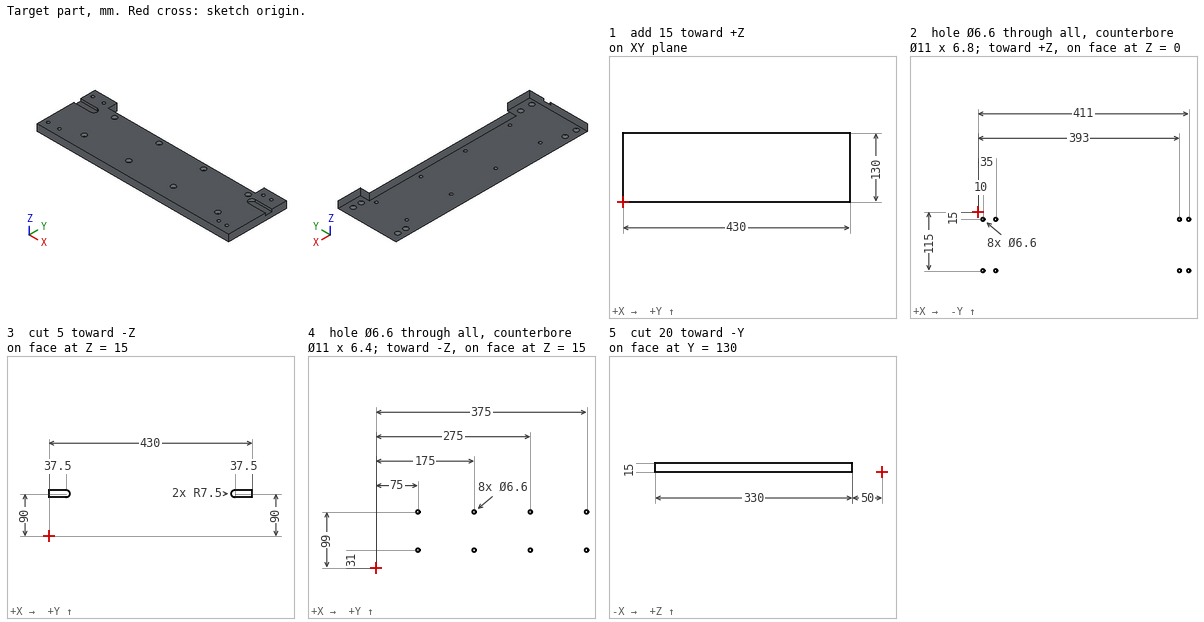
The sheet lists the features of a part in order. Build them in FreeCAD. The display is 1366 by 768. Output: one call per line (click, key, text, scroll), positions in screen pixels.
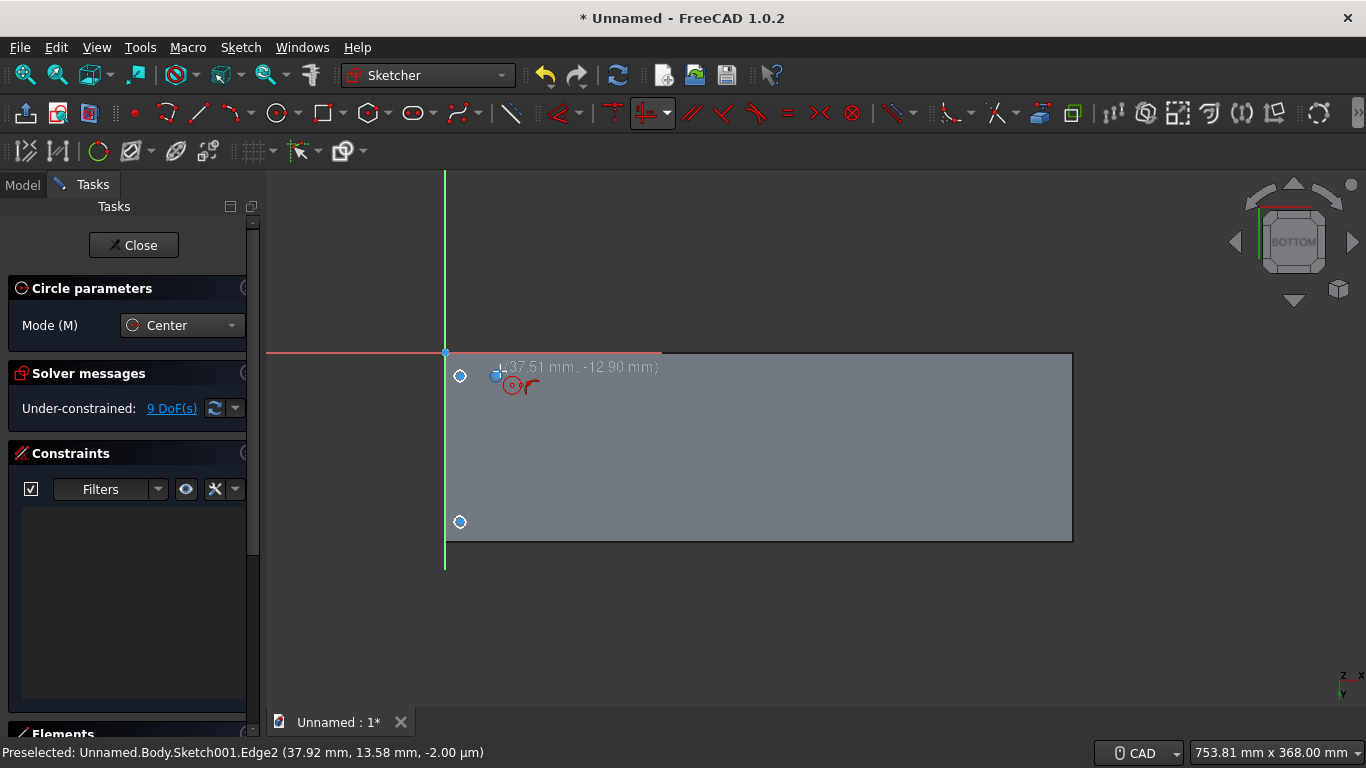
scroll(496, 521, up, 8)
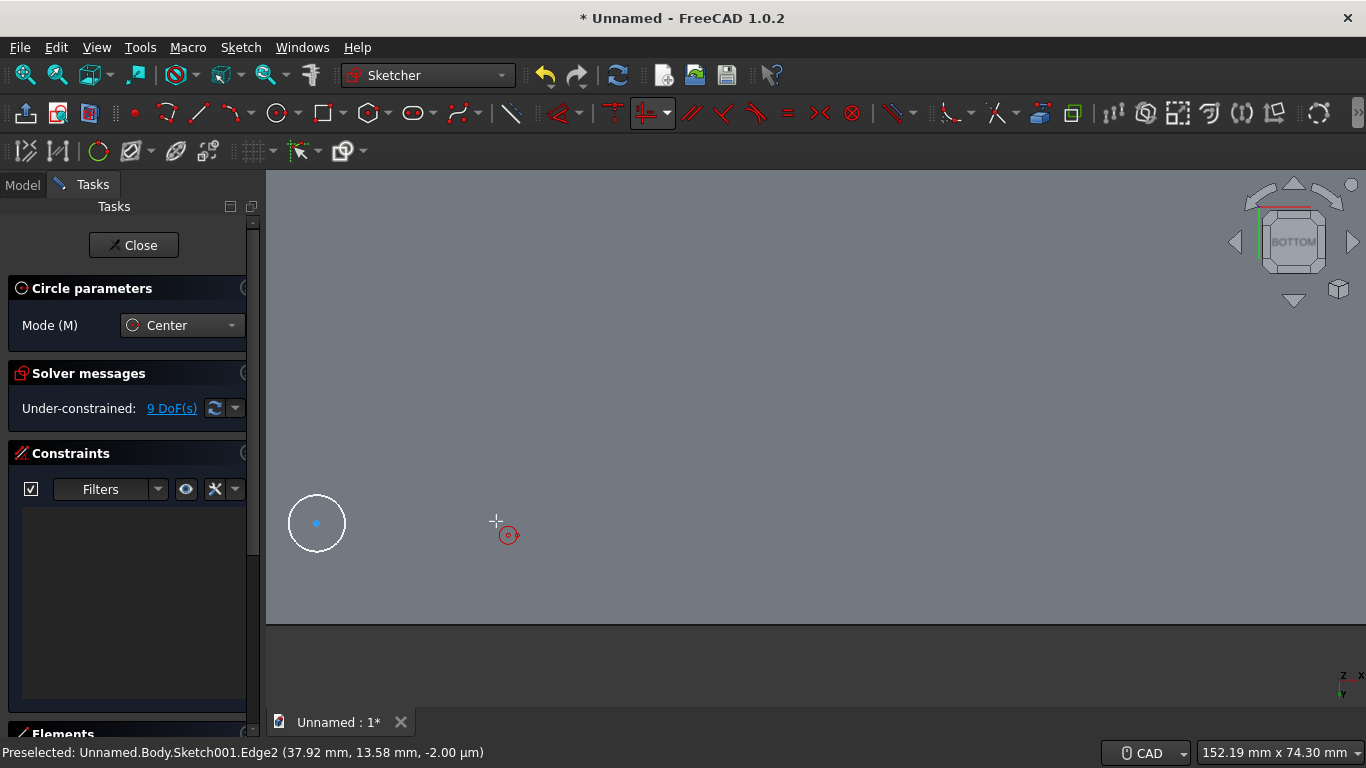
scroll(496, 521, down, 8)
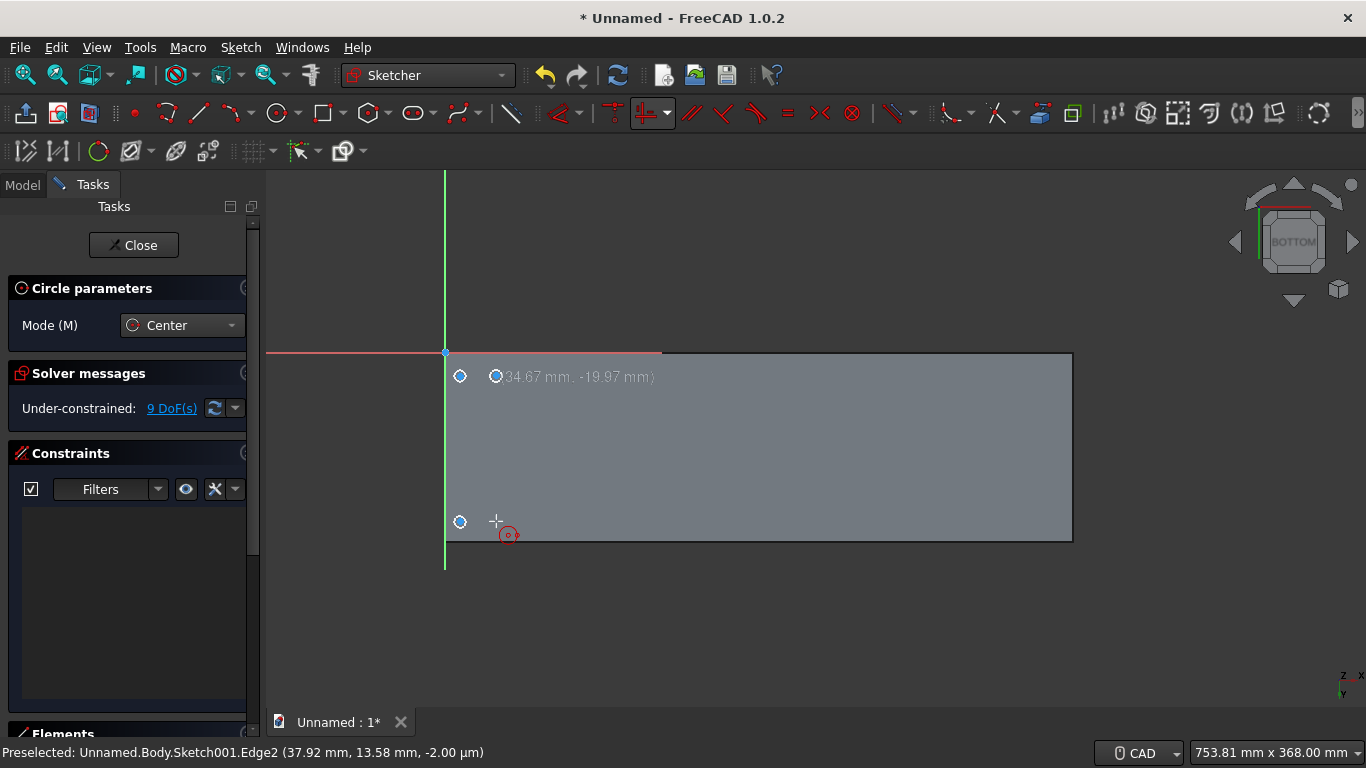
click(496, 521)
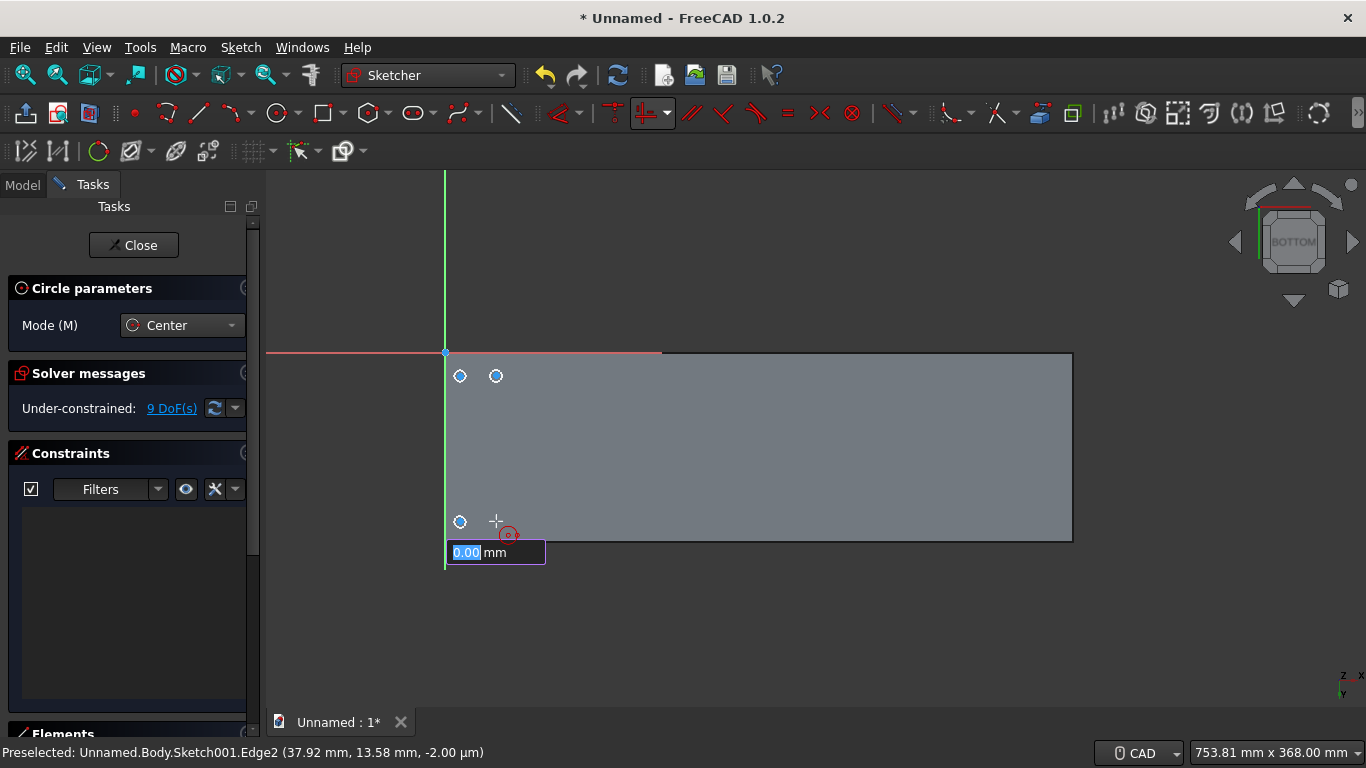
scroll(500, 517, up, 6)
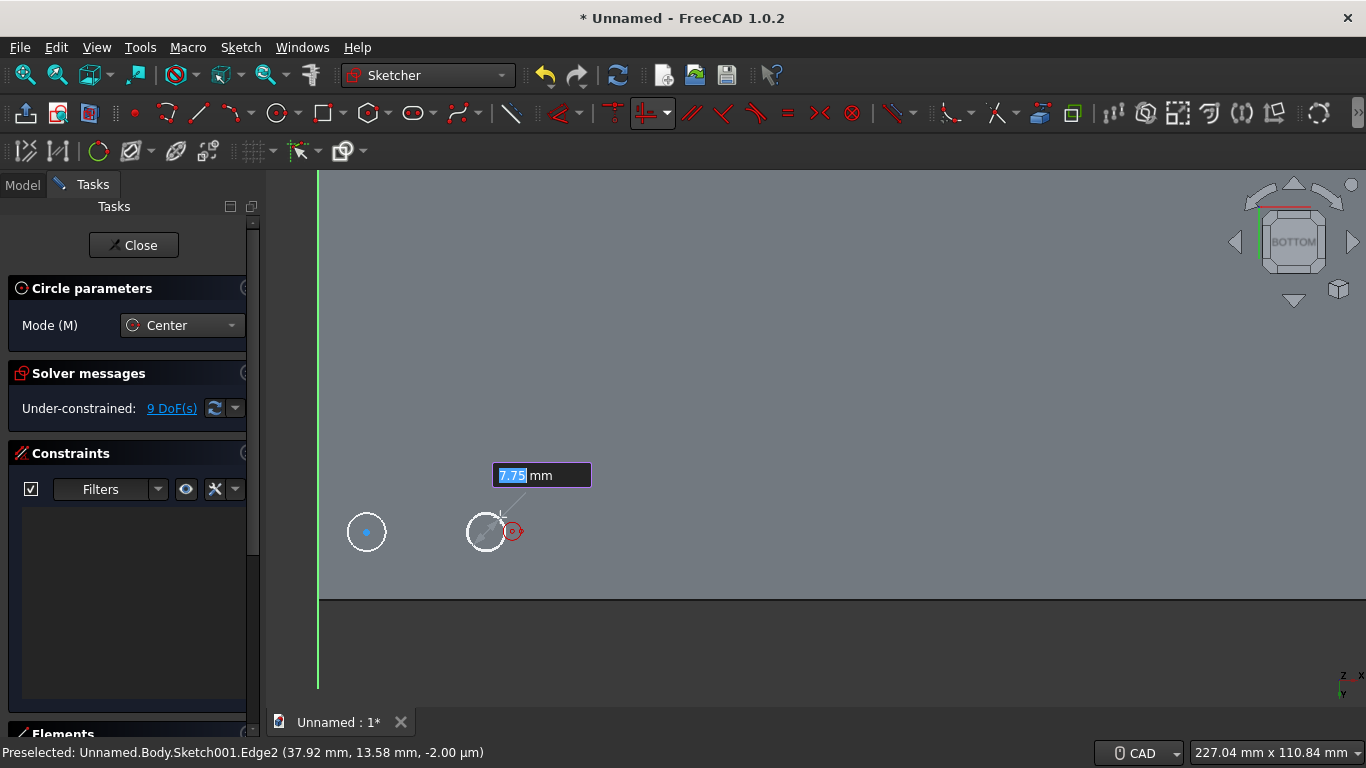
click(499, 516)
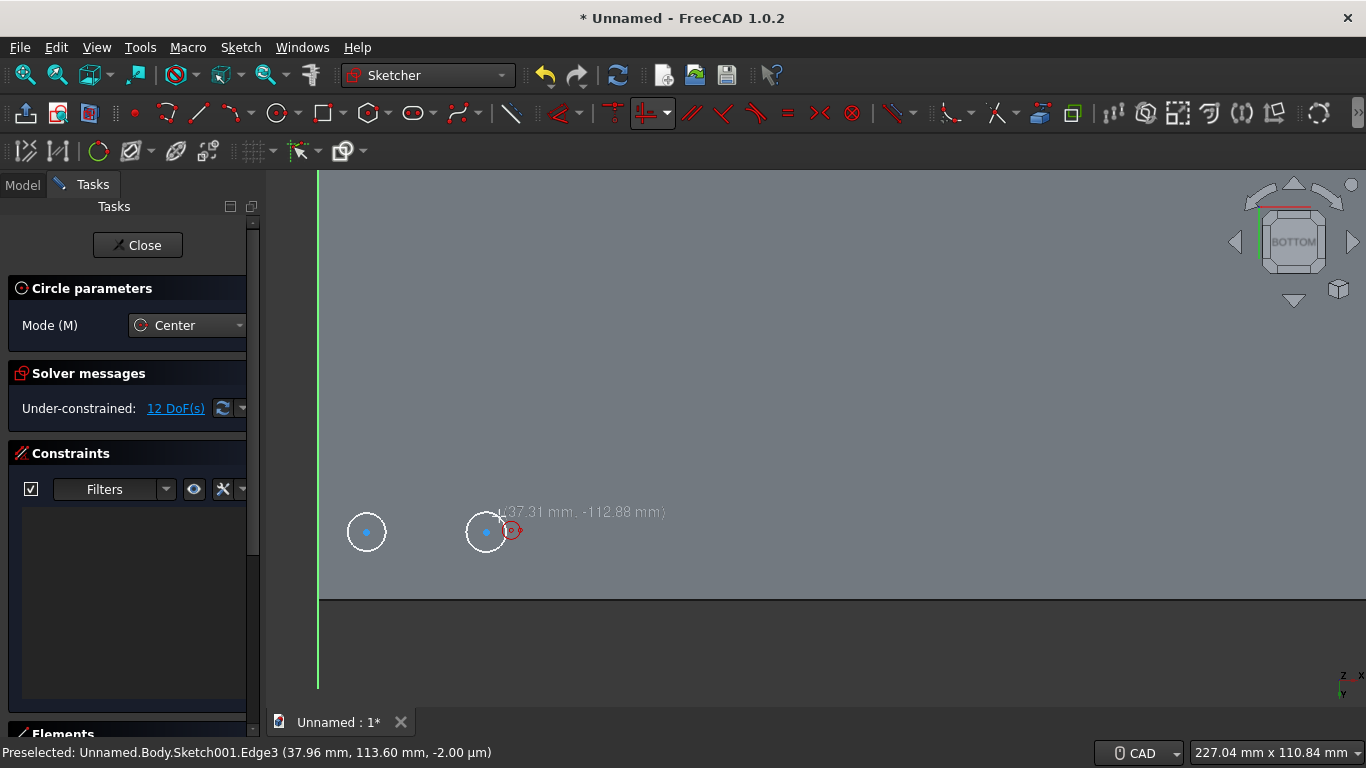
scroll(500, 517, down, 6)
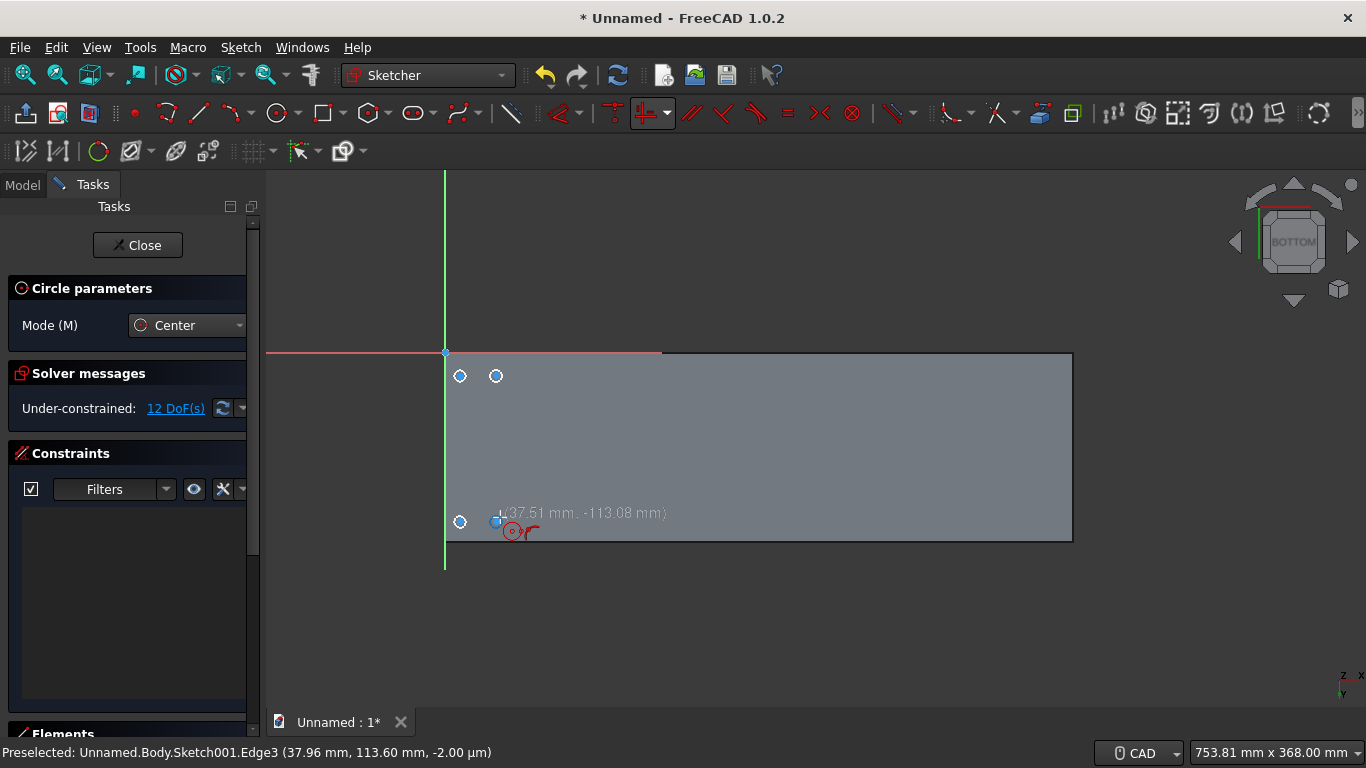
scroll(1019, 375, up, 8)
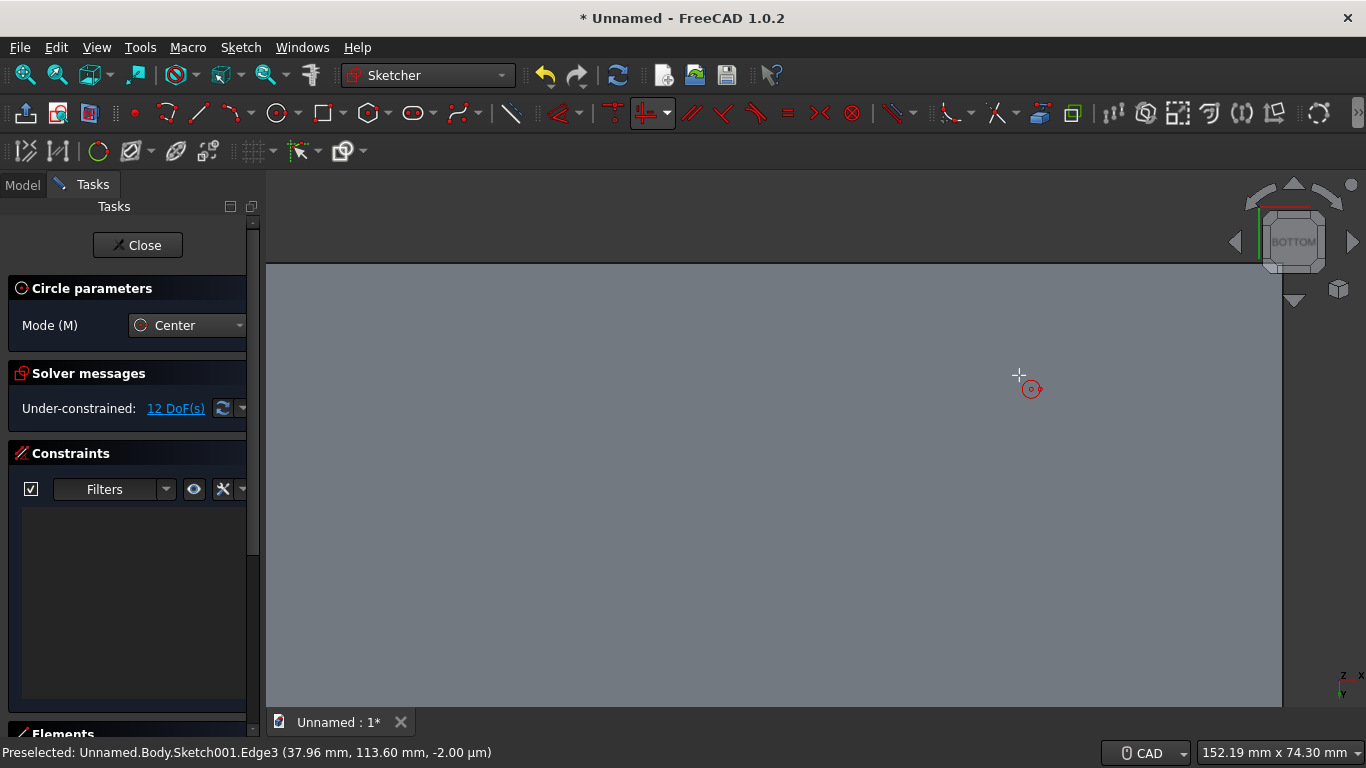
scroll(1019, 375, down, 8)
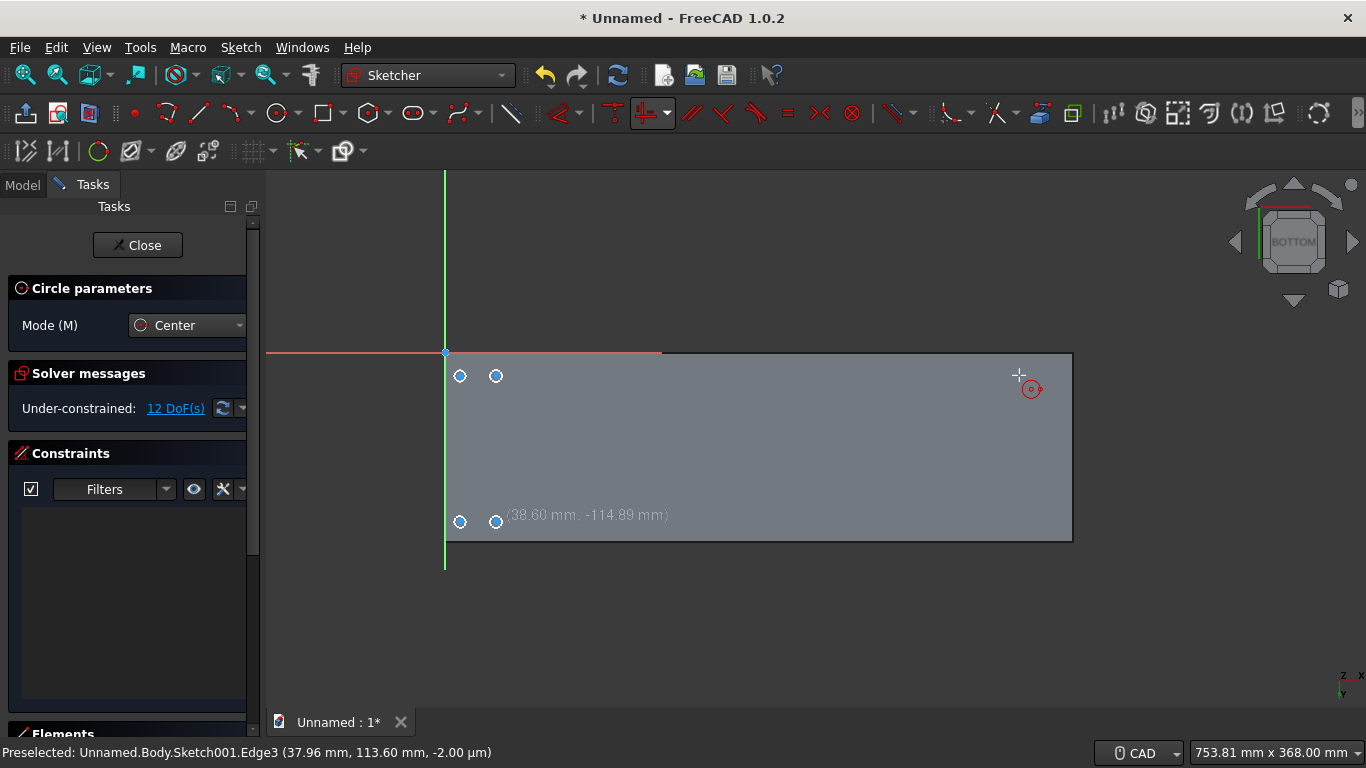
click(1019, 375)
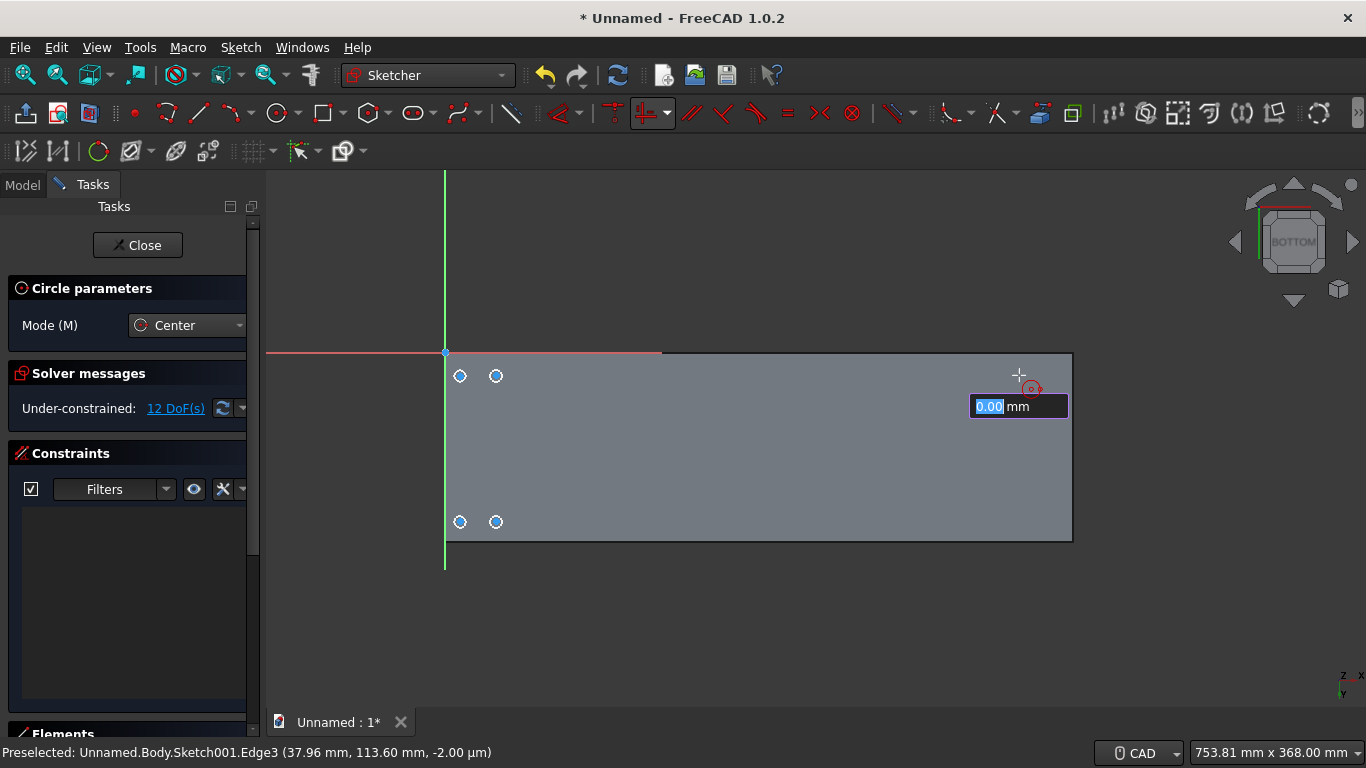
scroll(1022, 371, up, 6)